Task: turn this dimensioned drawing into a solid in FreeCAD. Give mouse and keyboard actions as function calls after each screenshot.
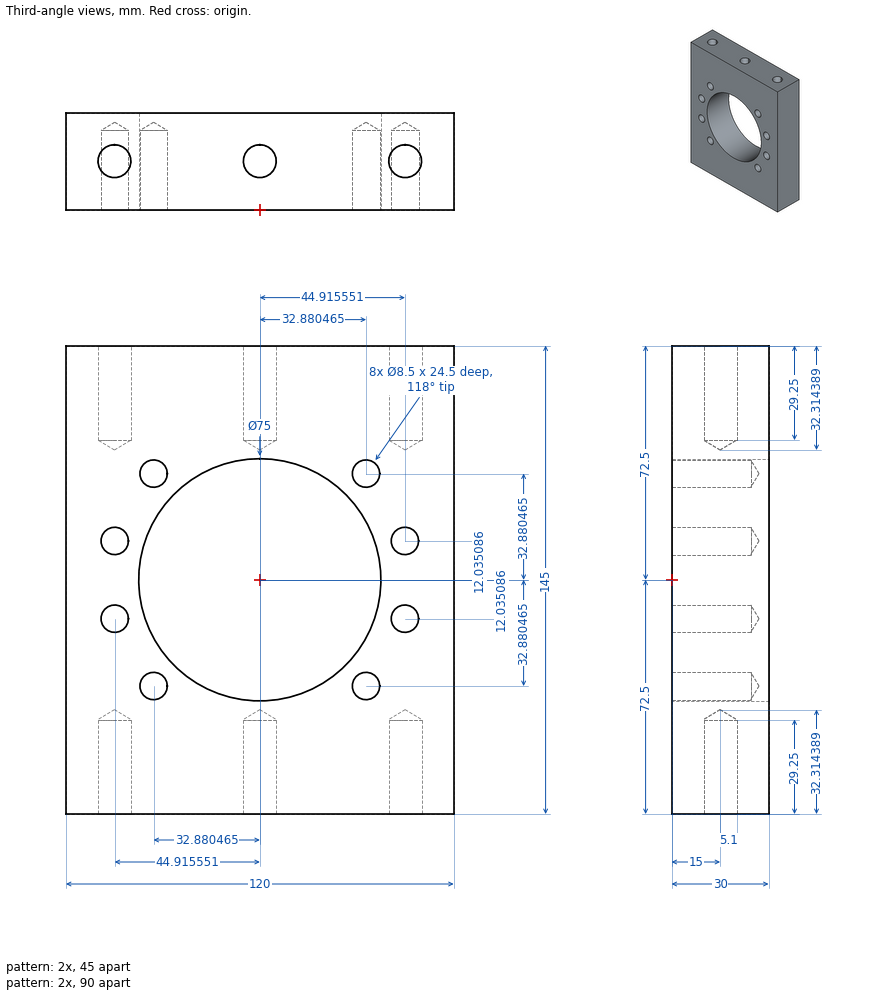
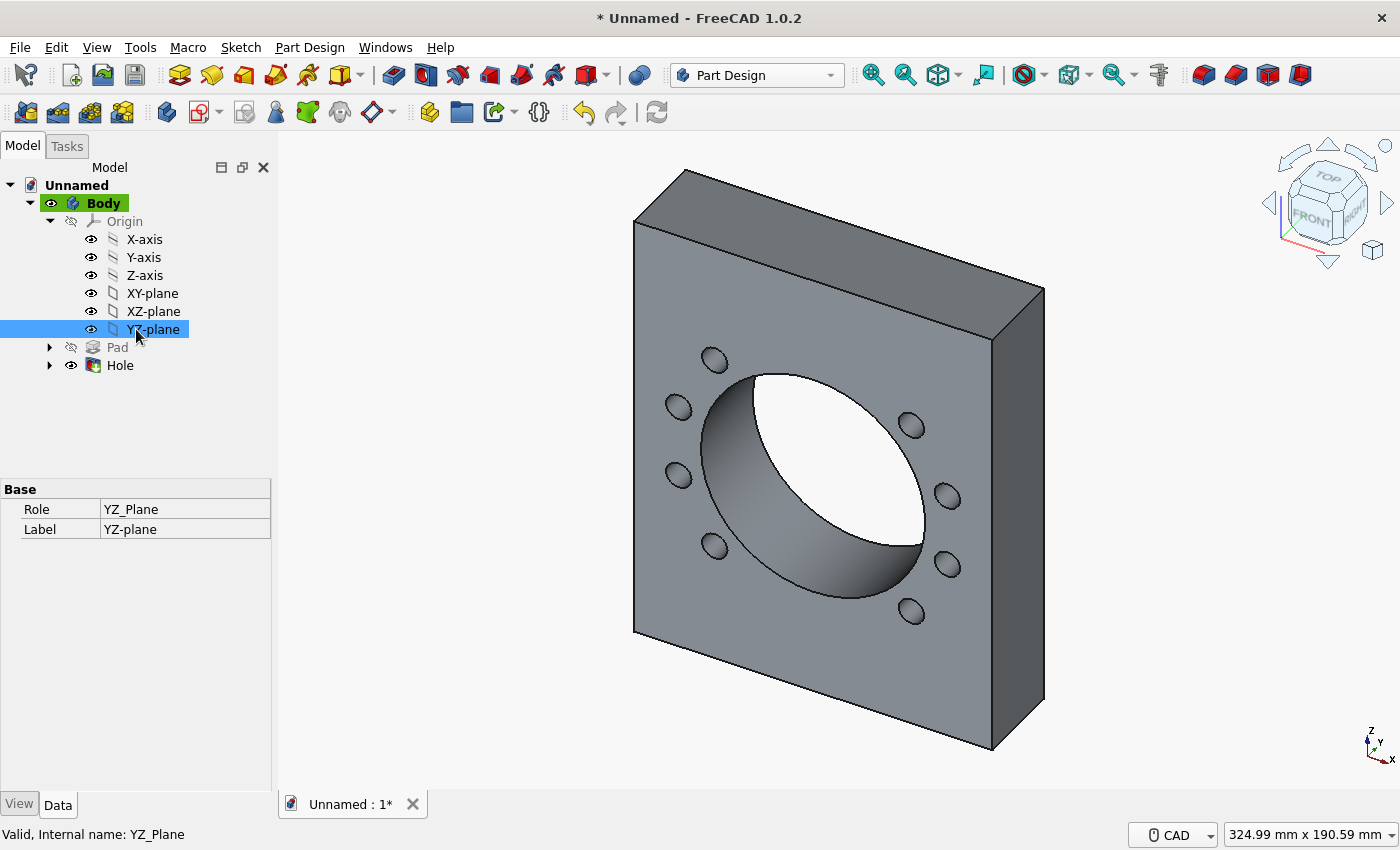
click(372, 112)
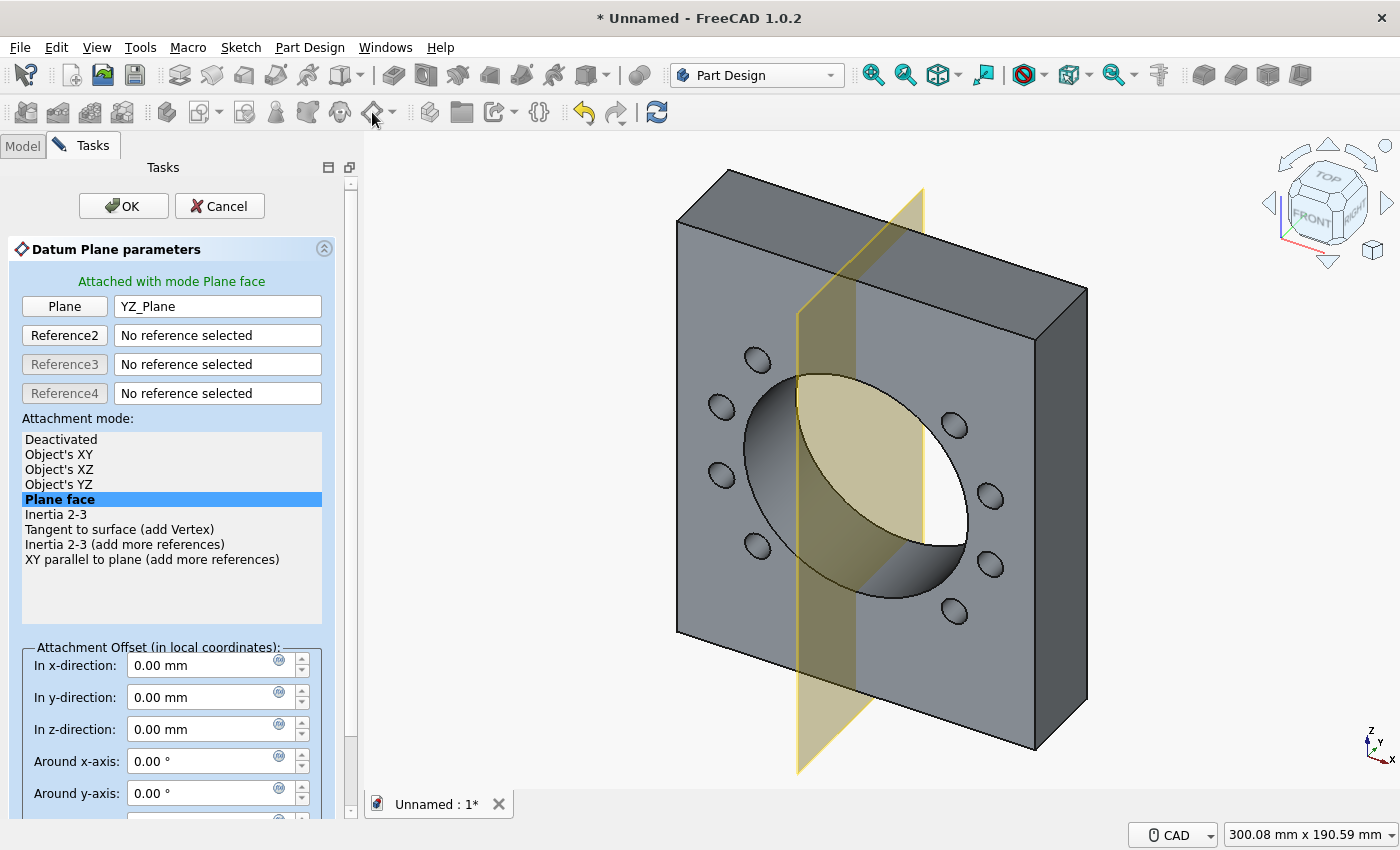
triple_click(210, 729)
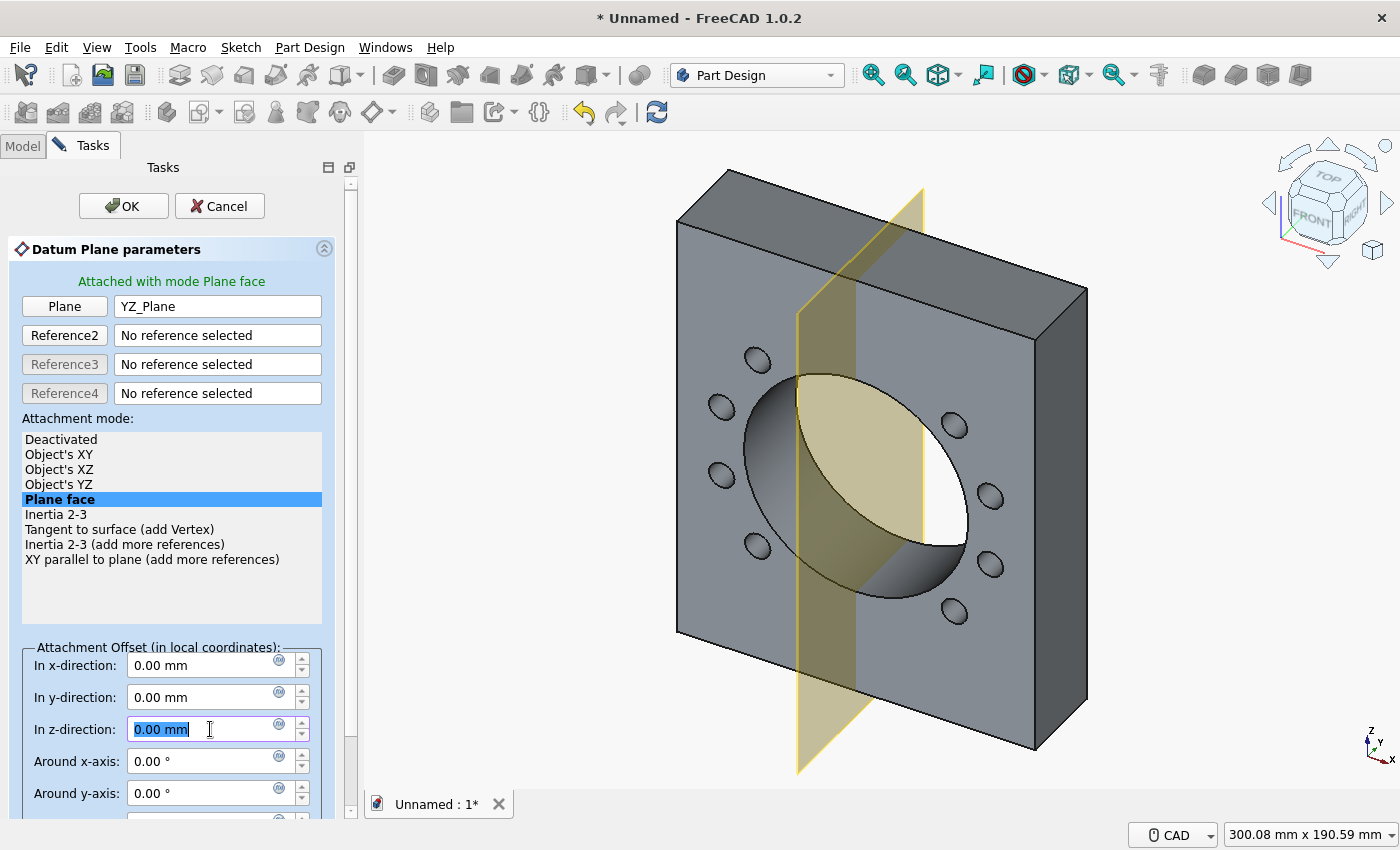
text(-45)
key(Tab)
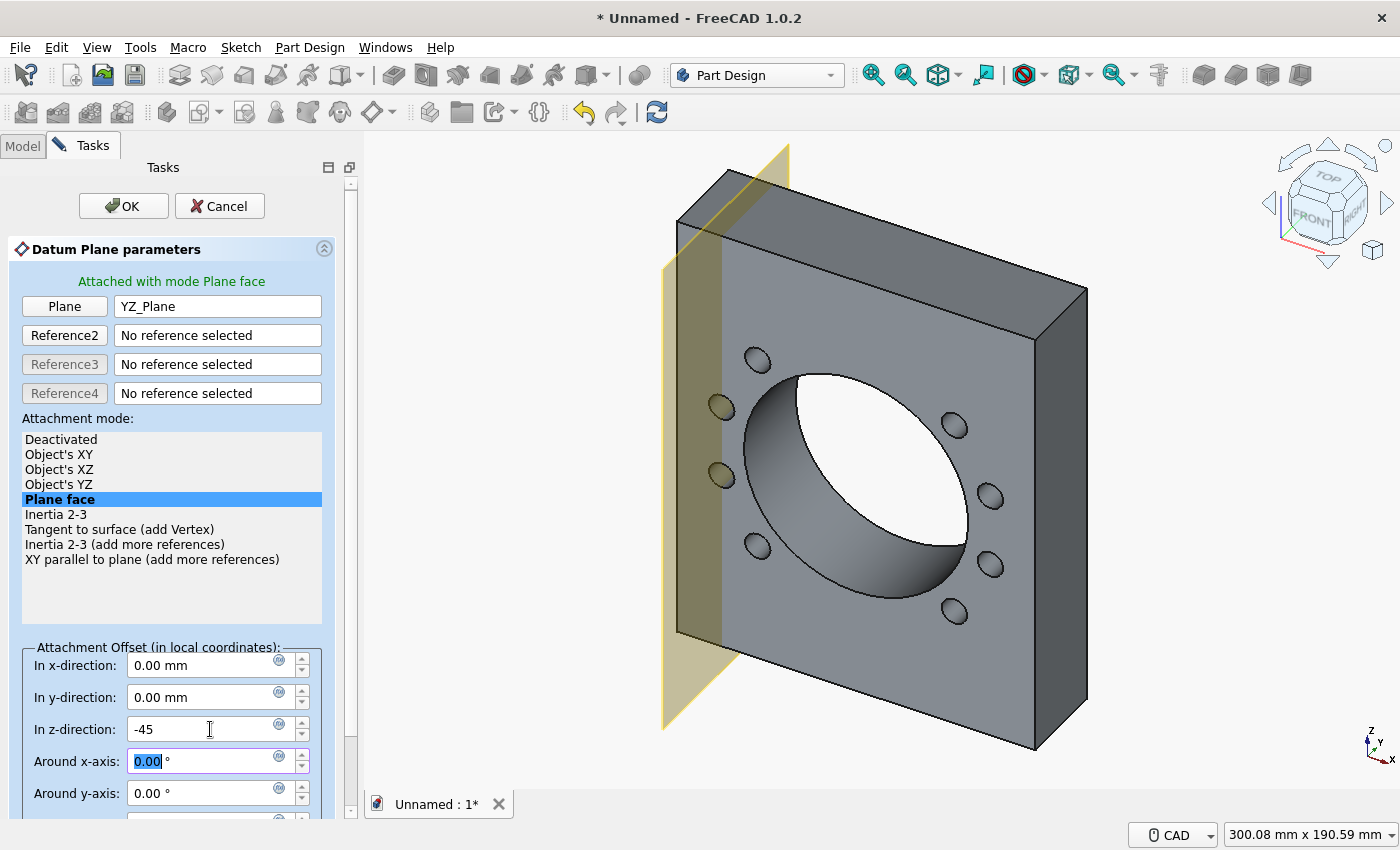
click(124, 206)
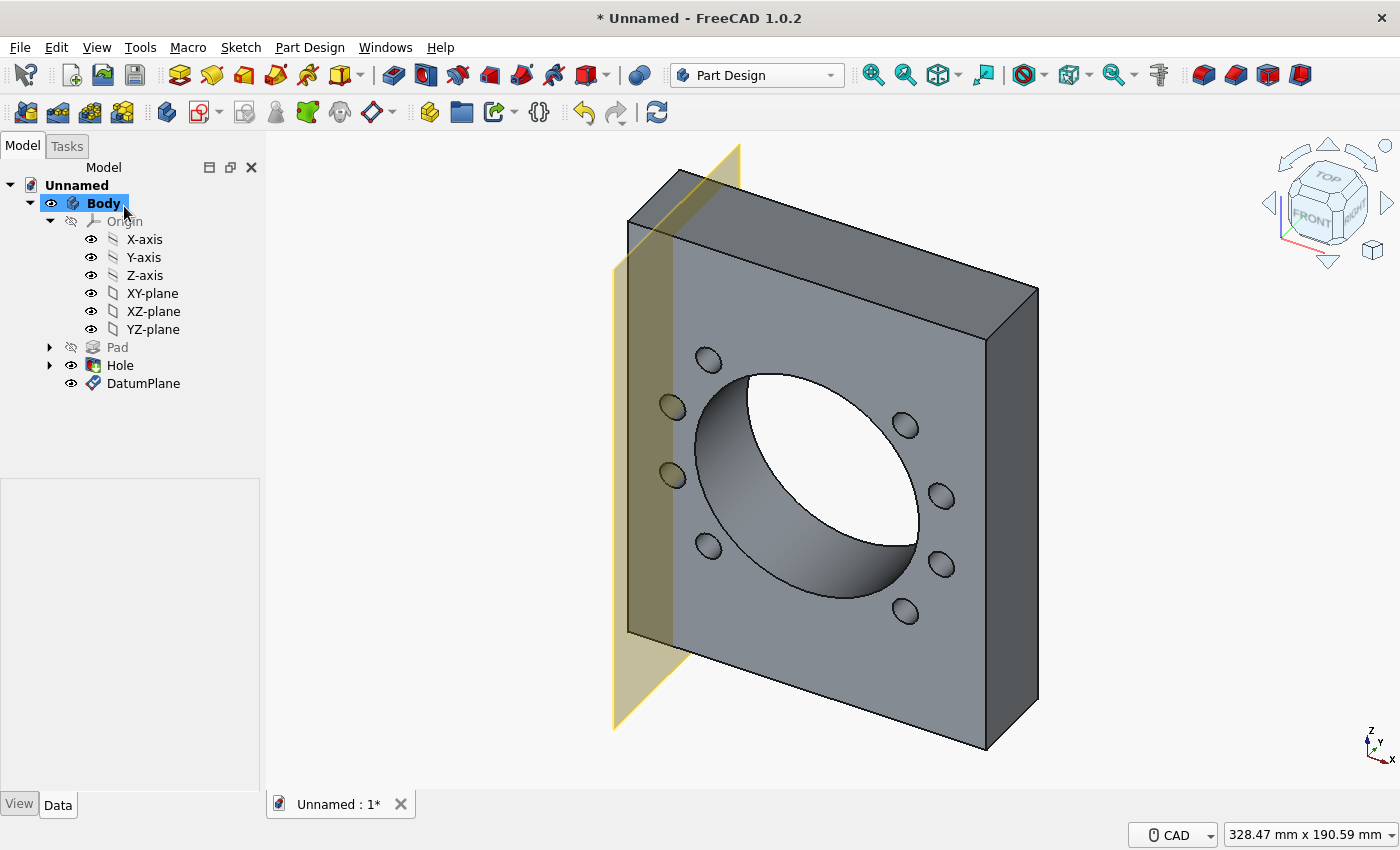
click(116, 383)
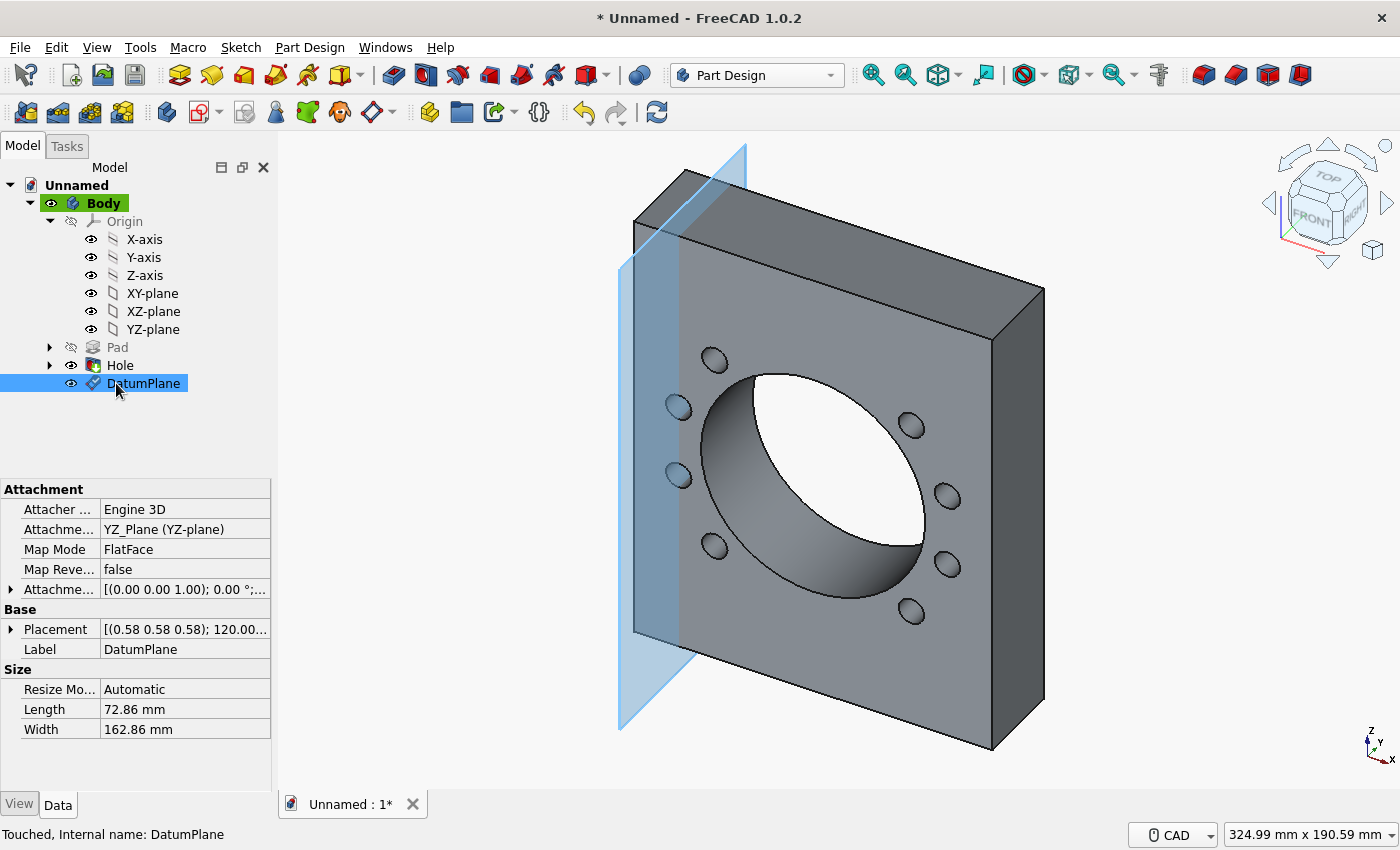
click(200, 112)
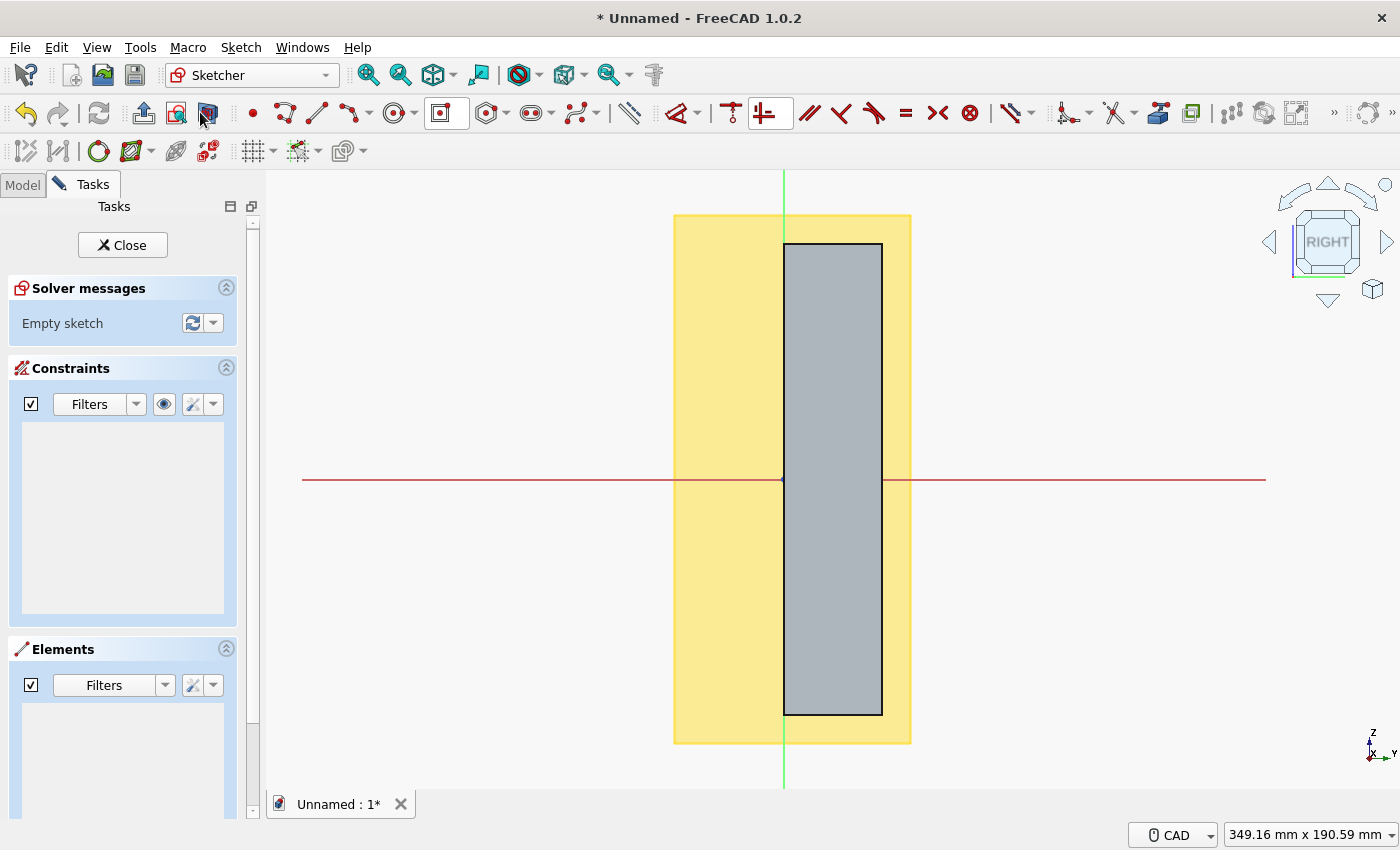
click(208, 114)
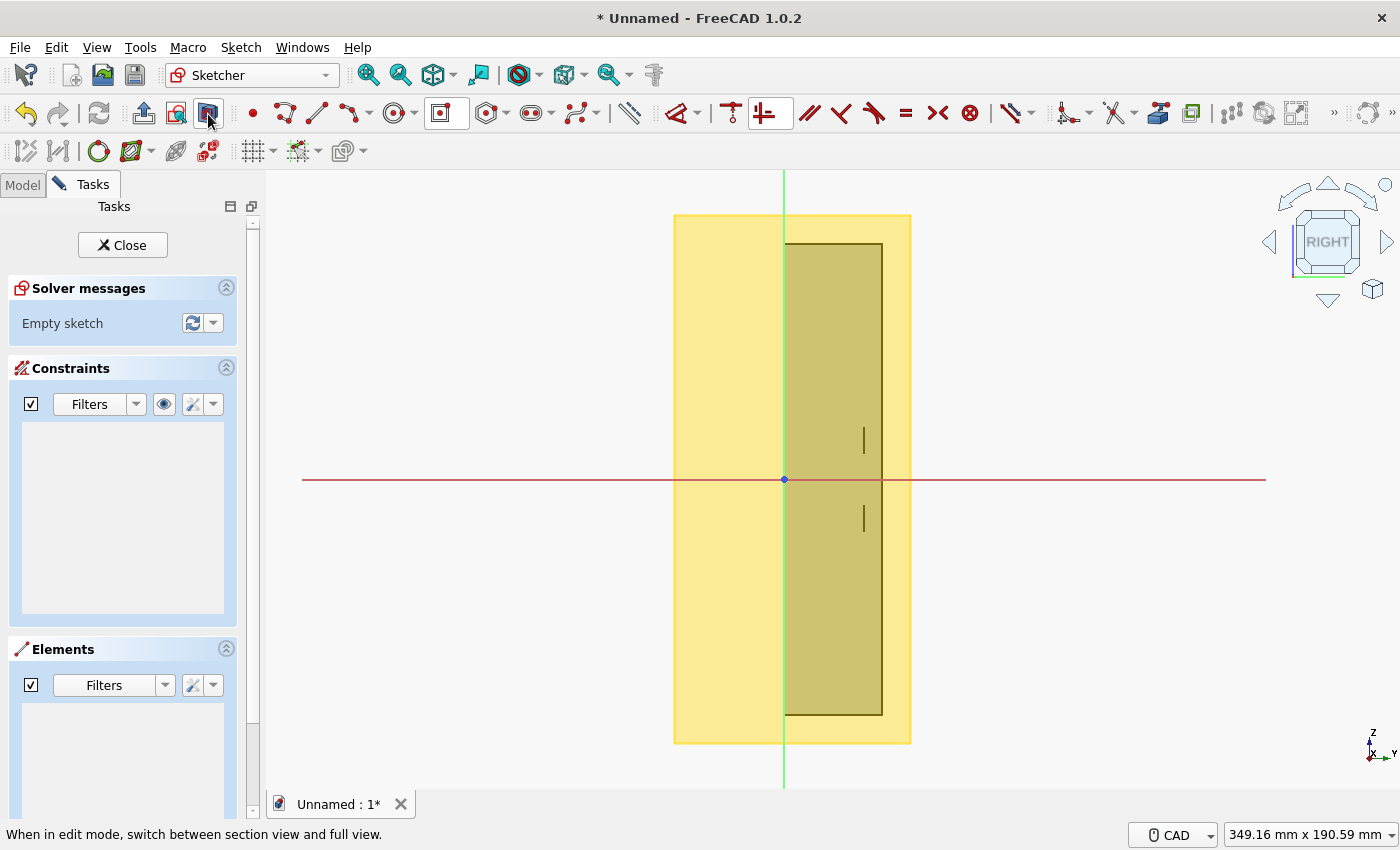
scroll(881, 740, up, 3)